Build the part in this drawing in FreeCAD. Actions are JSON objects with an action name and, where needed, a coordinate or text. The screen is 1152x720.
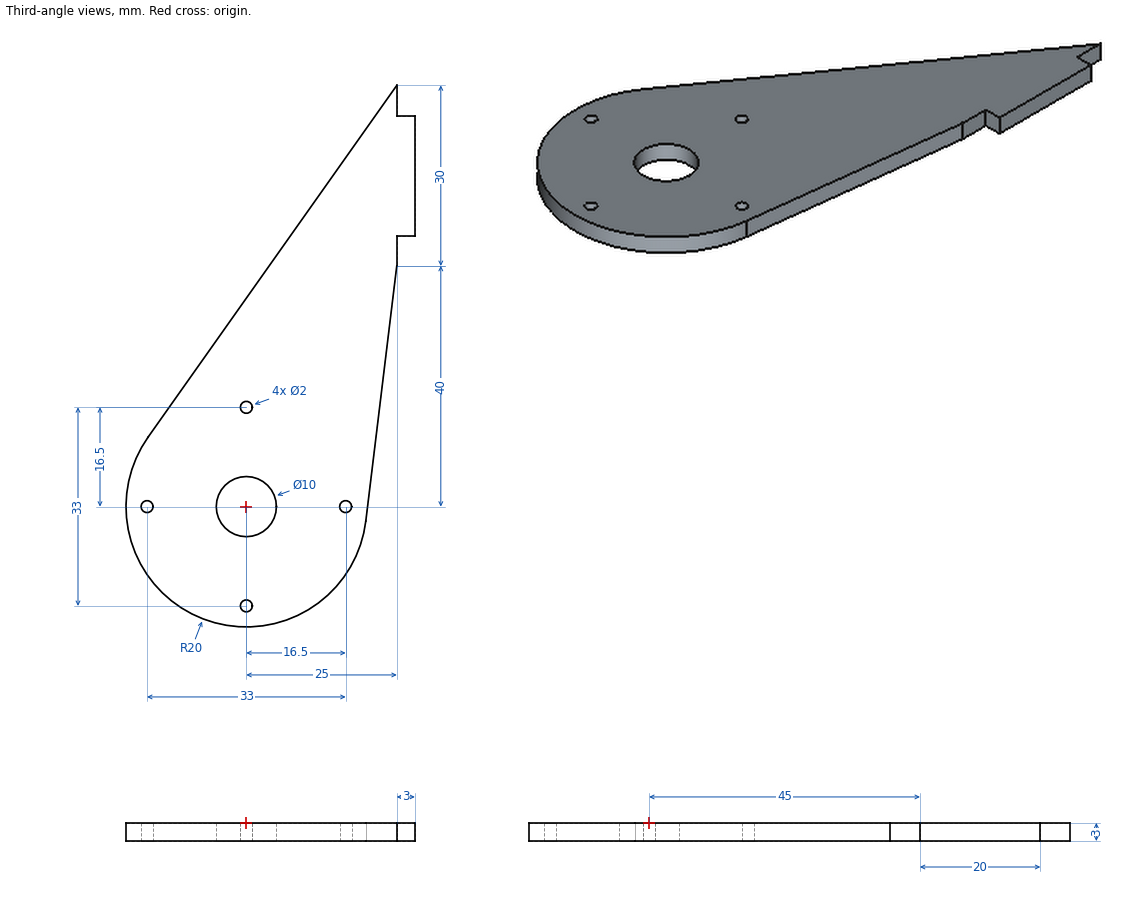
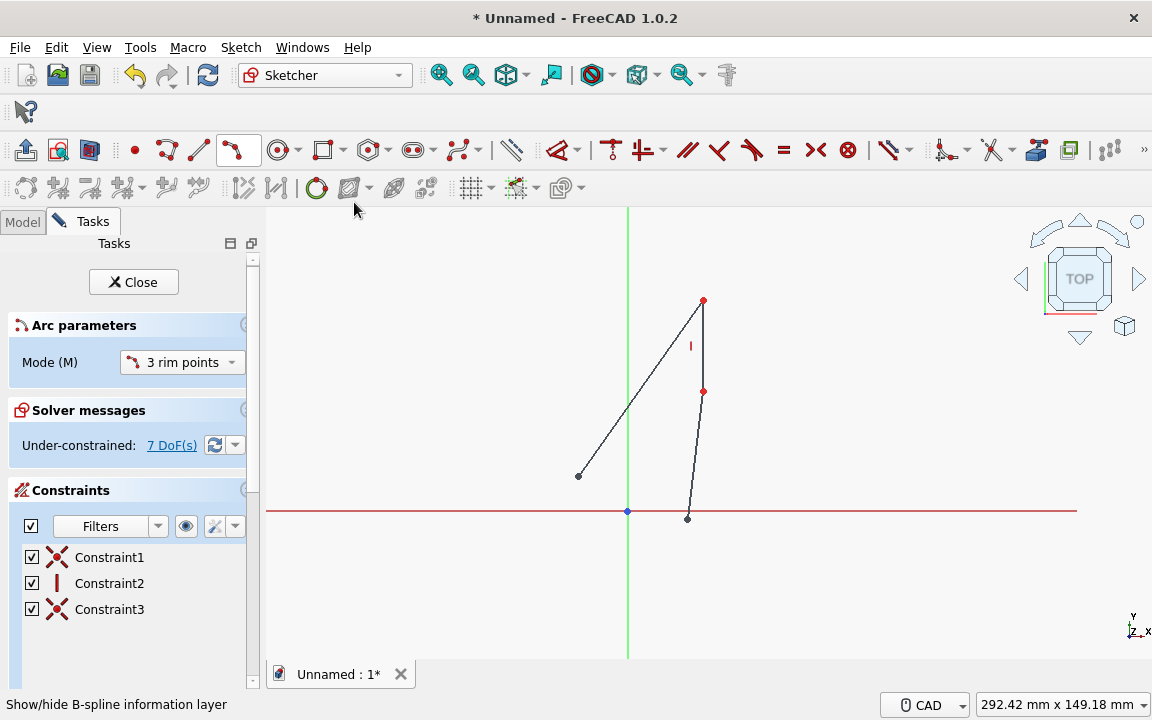
{"action": "left_click", "coordinate": [579, 477]}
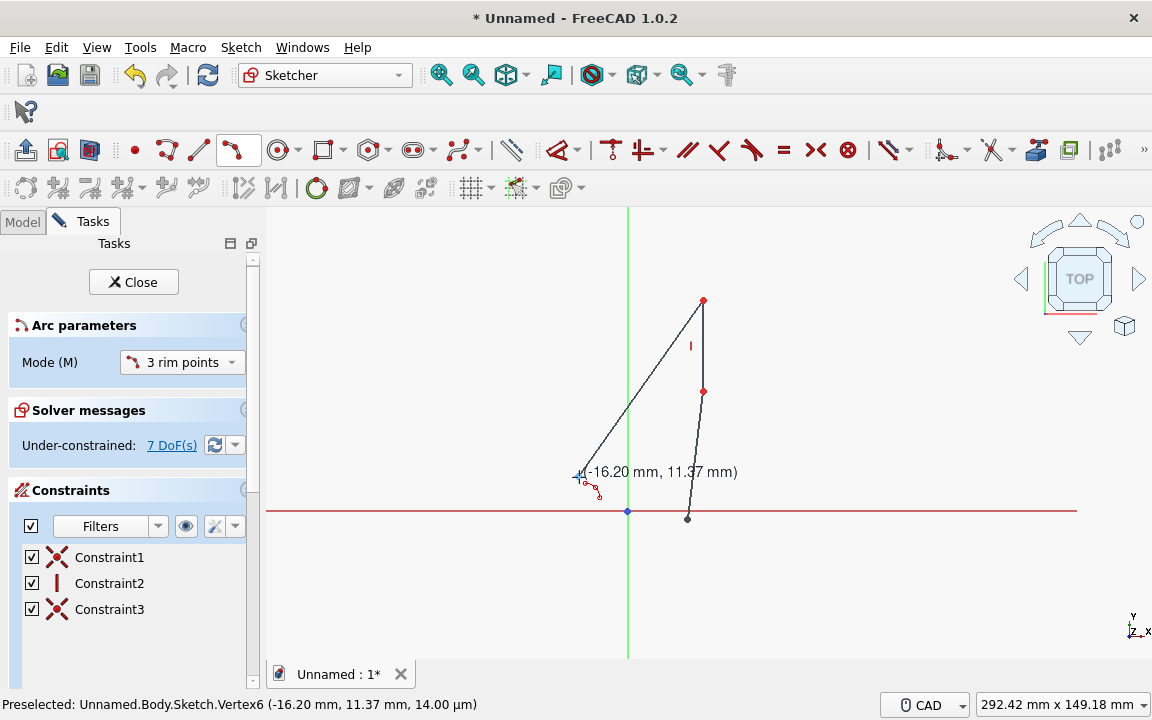
{"action": "scroll", "coordinate": [688, 519], "scroll_direction": "up", "scroll_amount": 4}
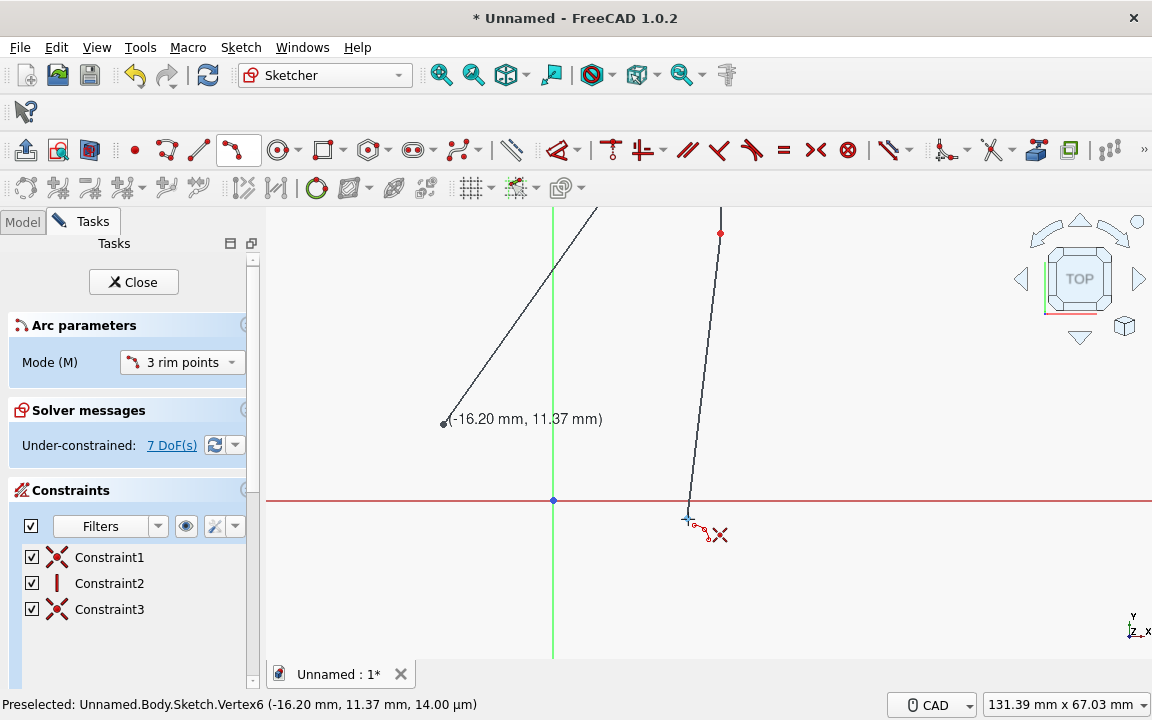
{"action": "left_click", "coordinate": [687, 518]}
{"action": "left_click", "coordinate": [505, 627]}
{"action": "key", "text": "Escape"}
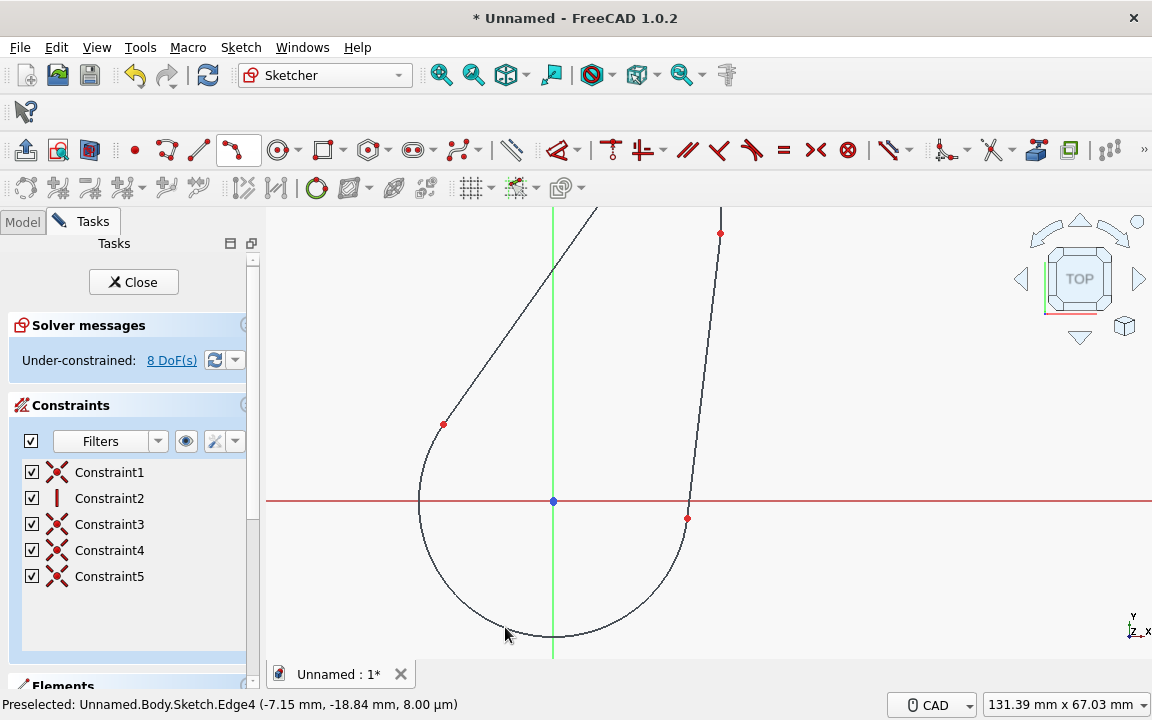
{"action": "left_click", "coordinate": [697, 433]}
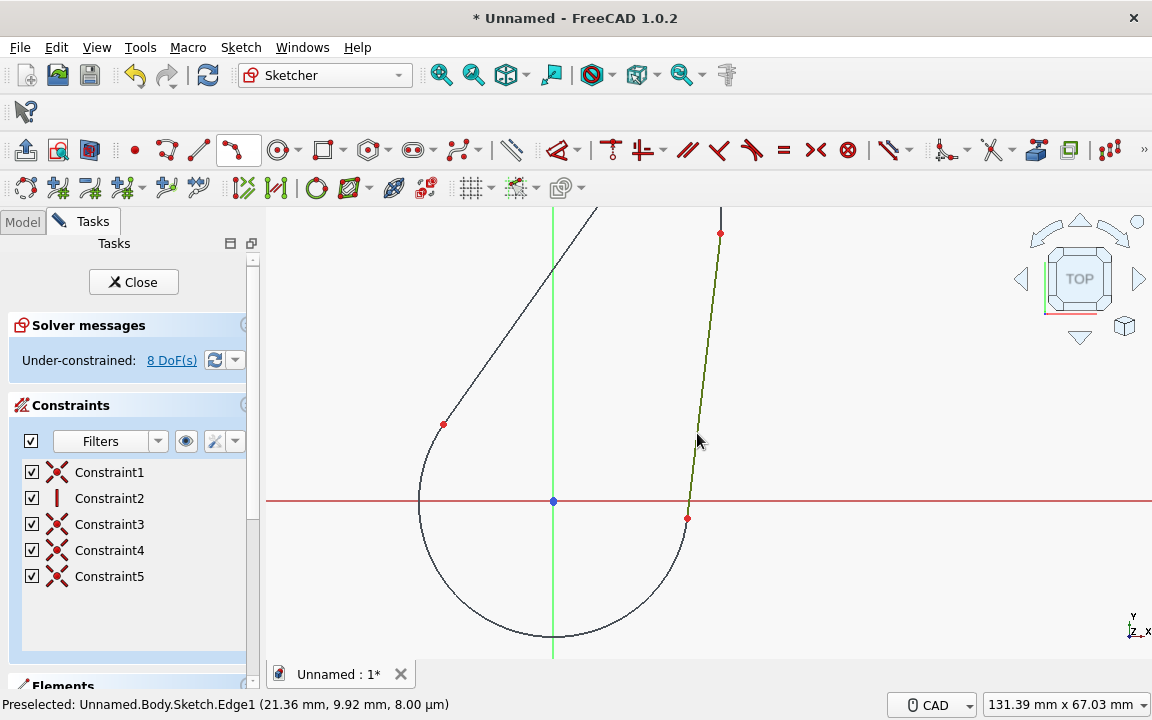
{"action": "left_click", "coordinate": [434, 564]}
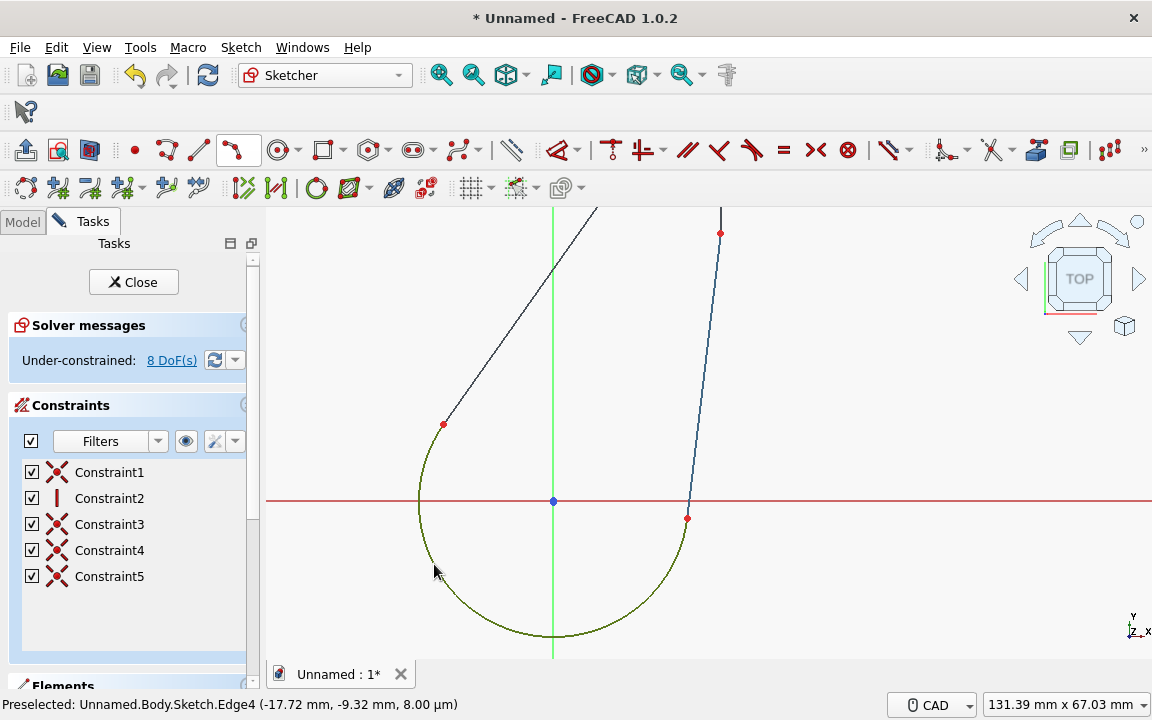
{"action": "left_click", "coordinate": [752, 150]}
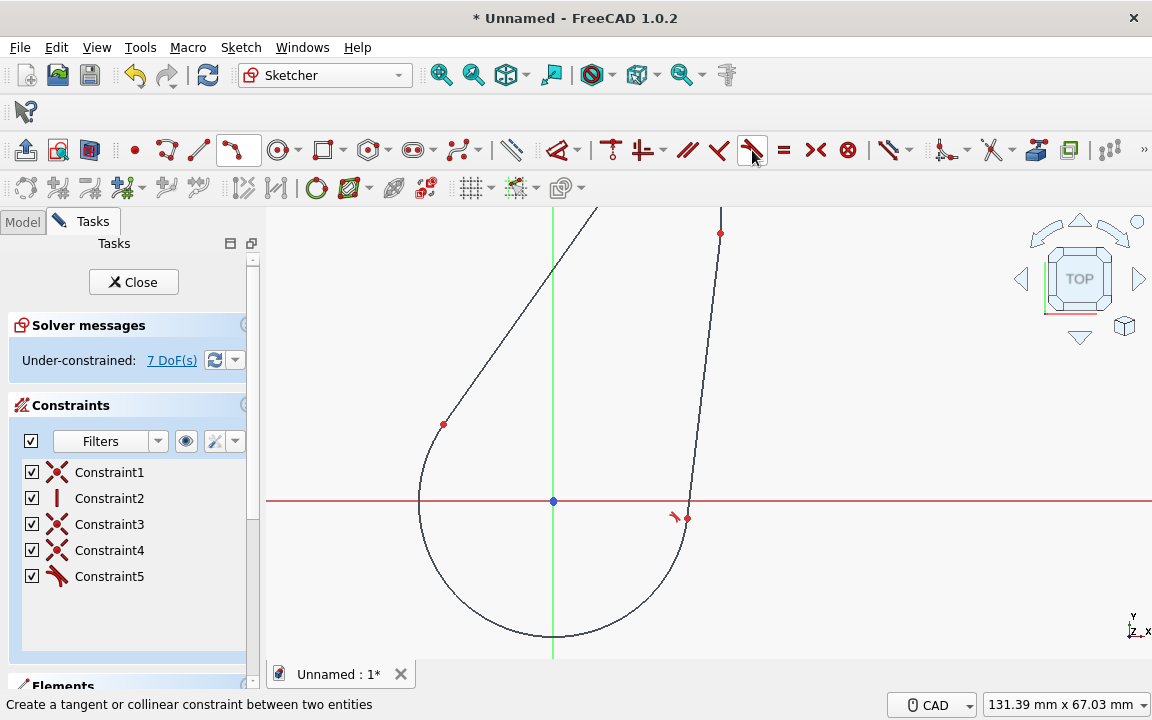
{"action": "left_click", "coordinate": [527, 307]}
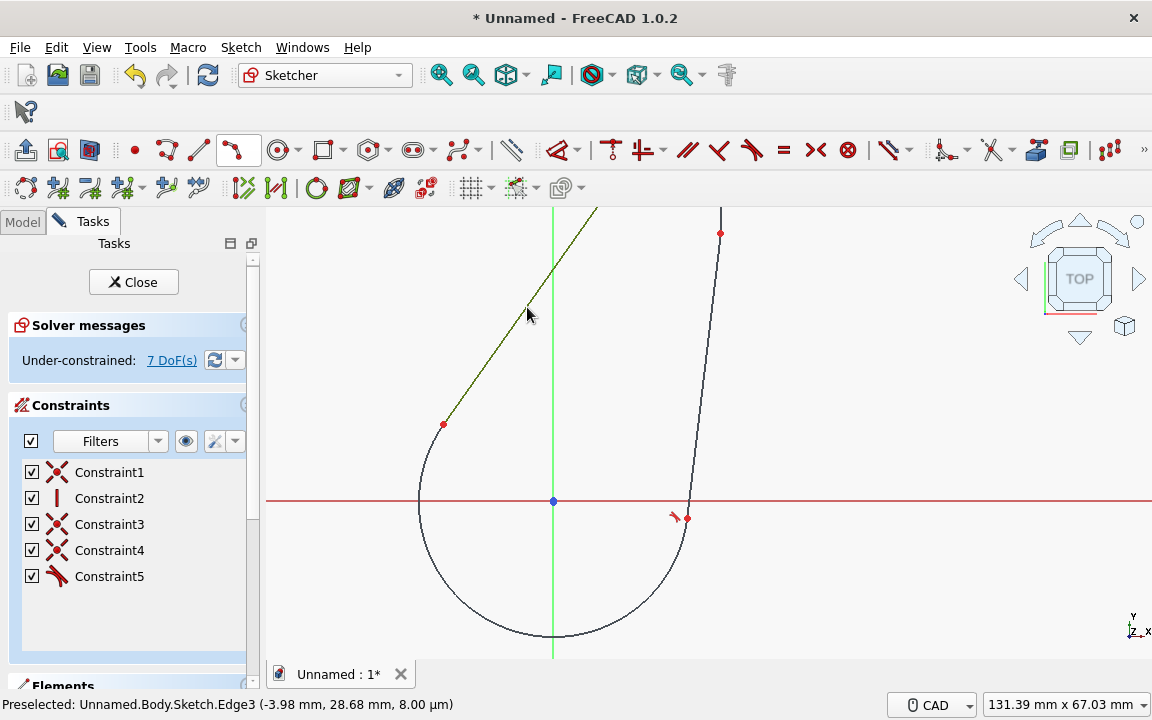
{"action": "left_click", "coordinate": [434, 564]}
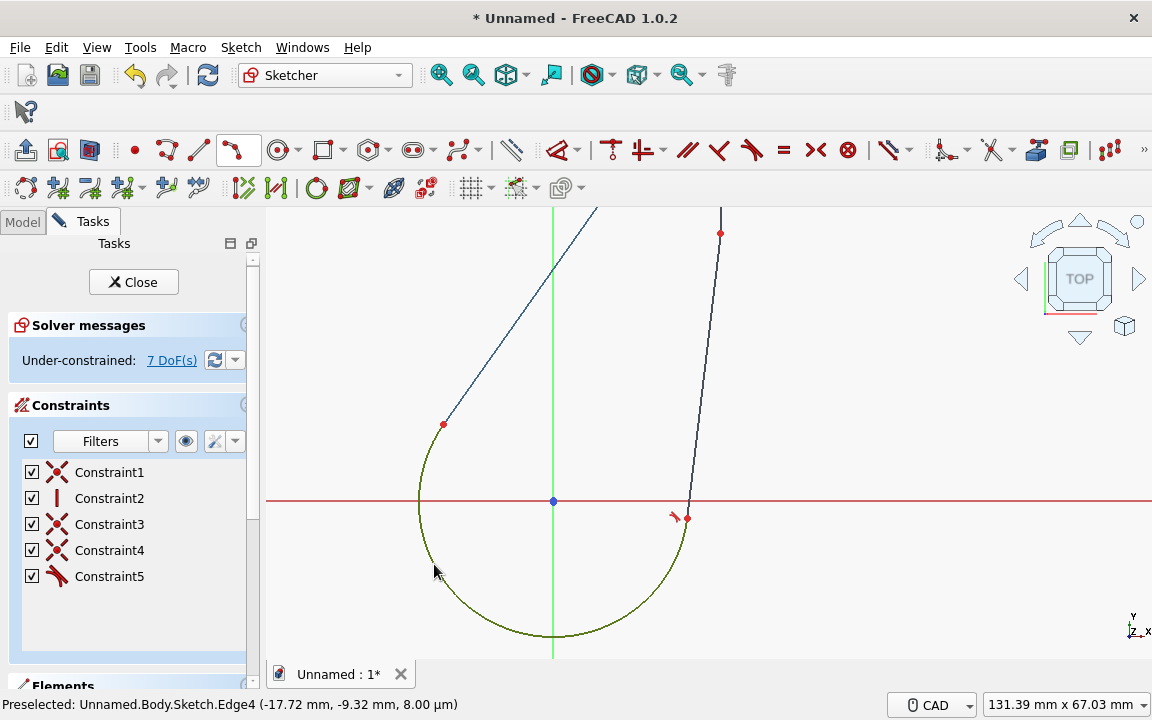
{"action": "left_click", "coordinate": [752, 150]}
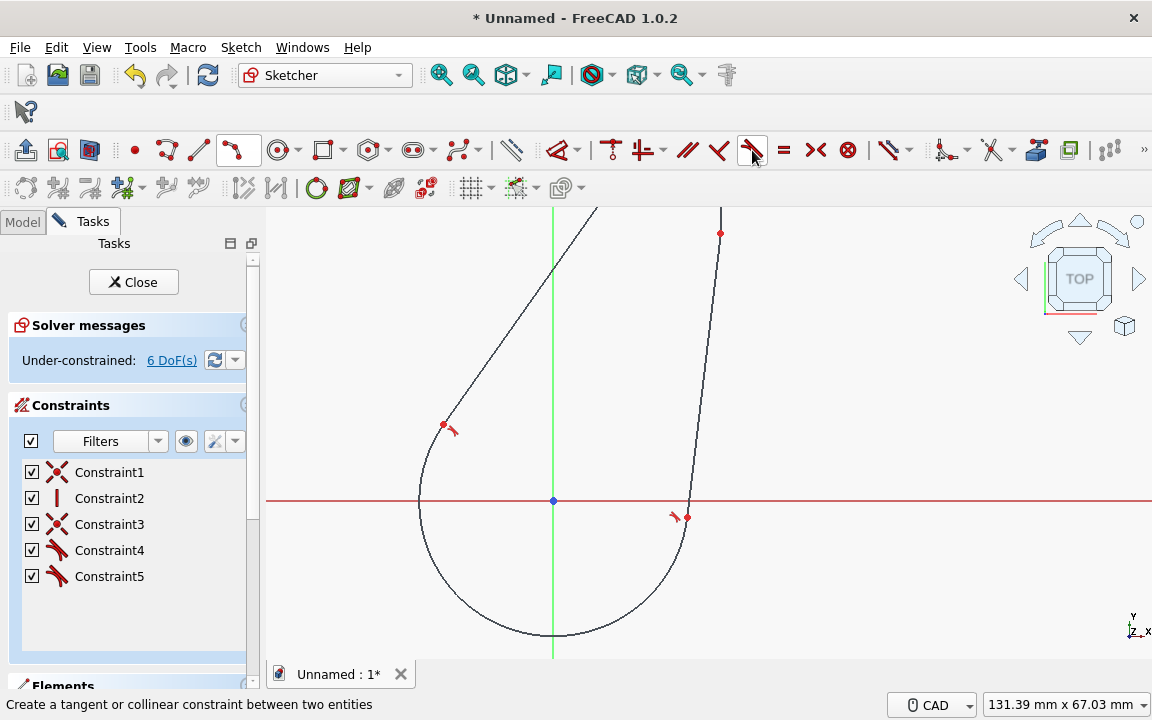
{"action": "left_click_drag", "start_coordinate": [543, 491], "coordinate": [564, 512]}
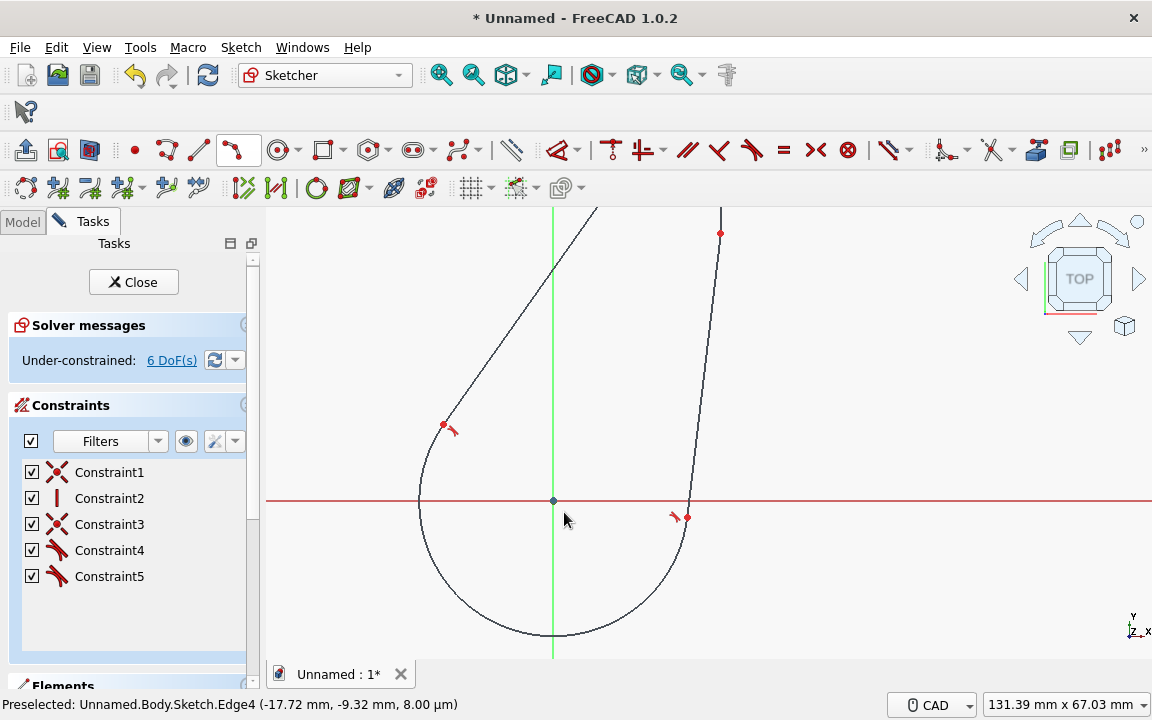
{"action": "left_click", "coordinate": [612, 150]}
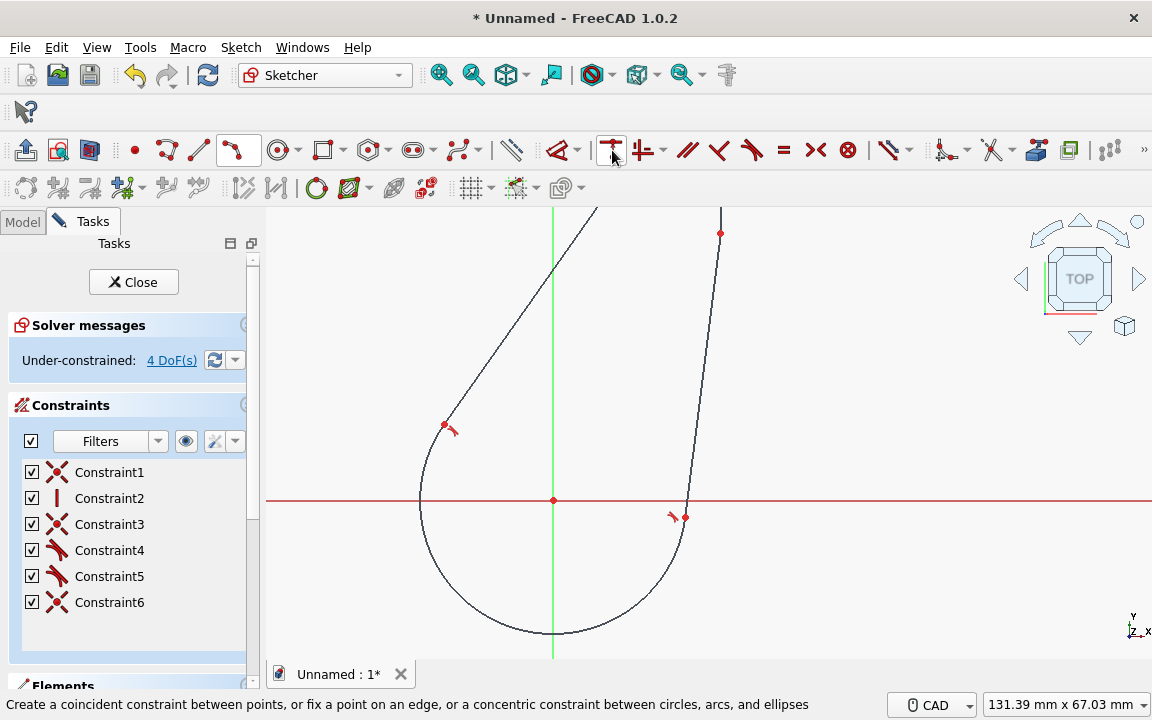
{"action": "left_click", "coordinate": [558, 150]}